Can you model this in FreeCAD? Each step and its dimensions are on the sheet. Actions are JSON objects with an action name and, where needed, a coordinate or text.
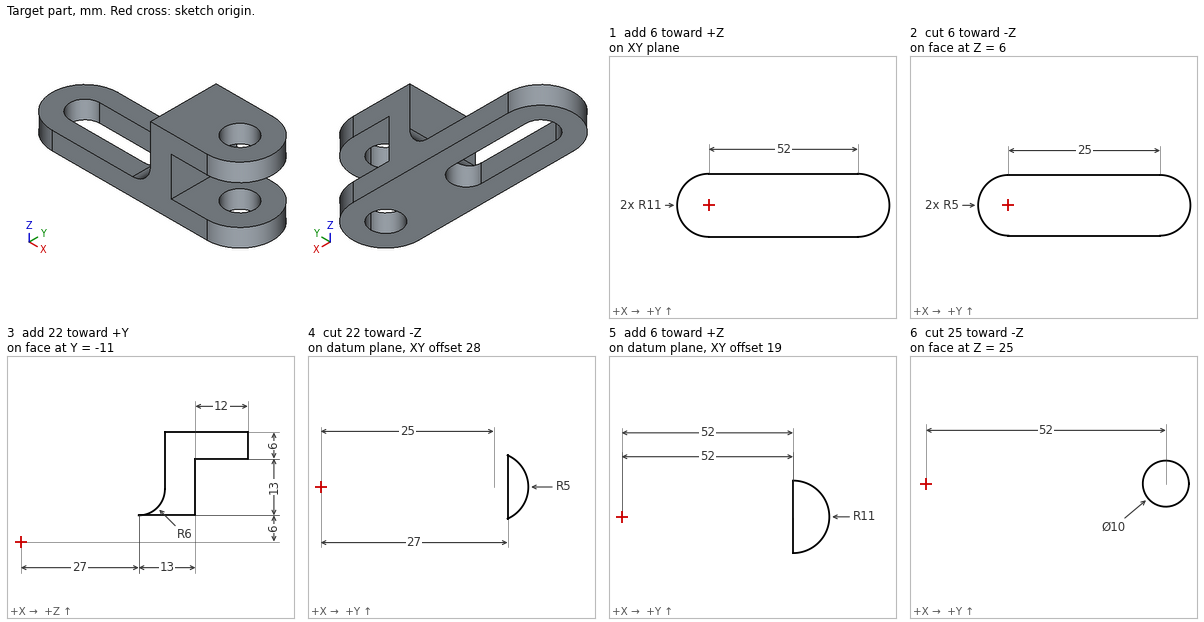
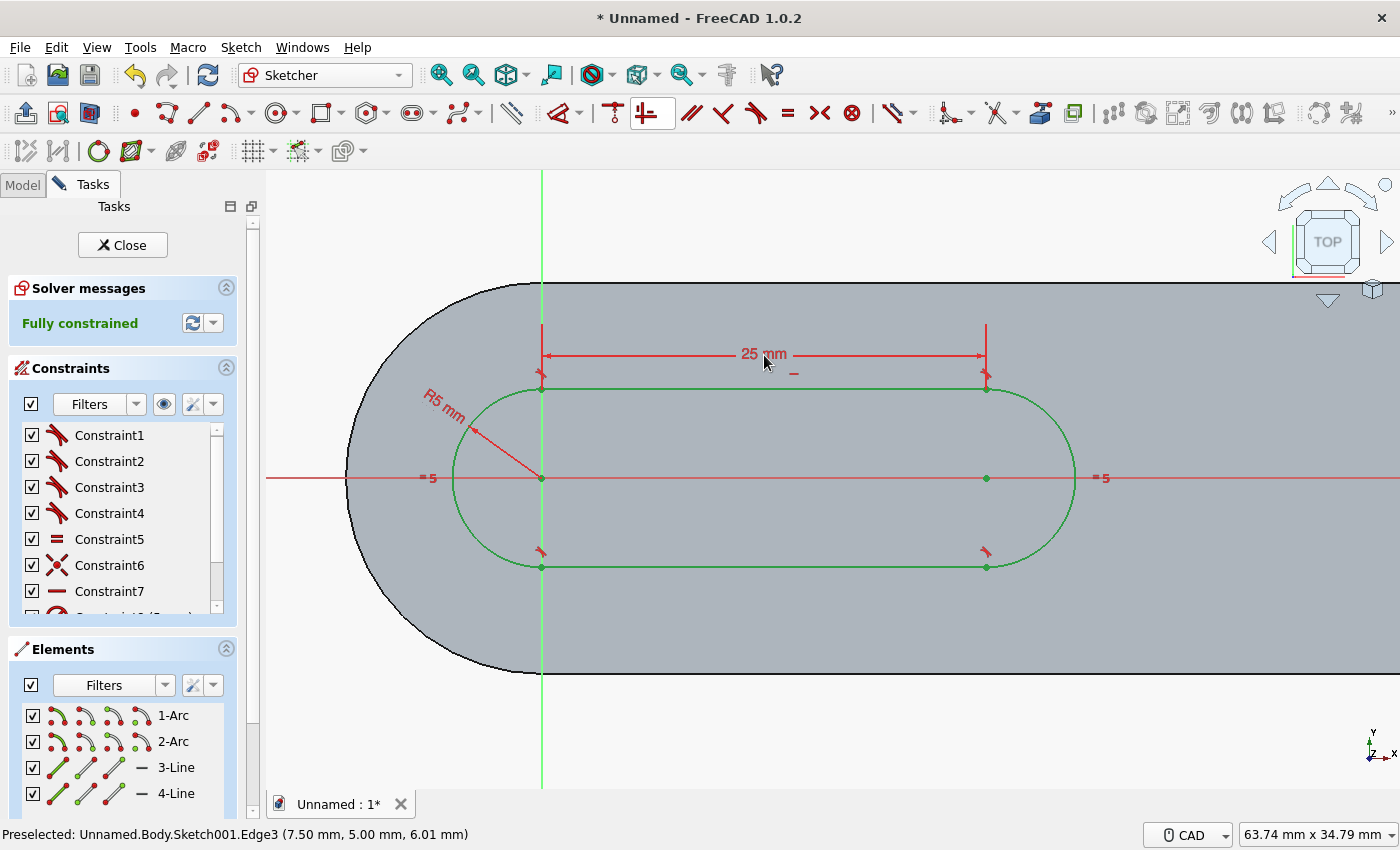
{"action": "left_click", "coordinate": [123, 245]}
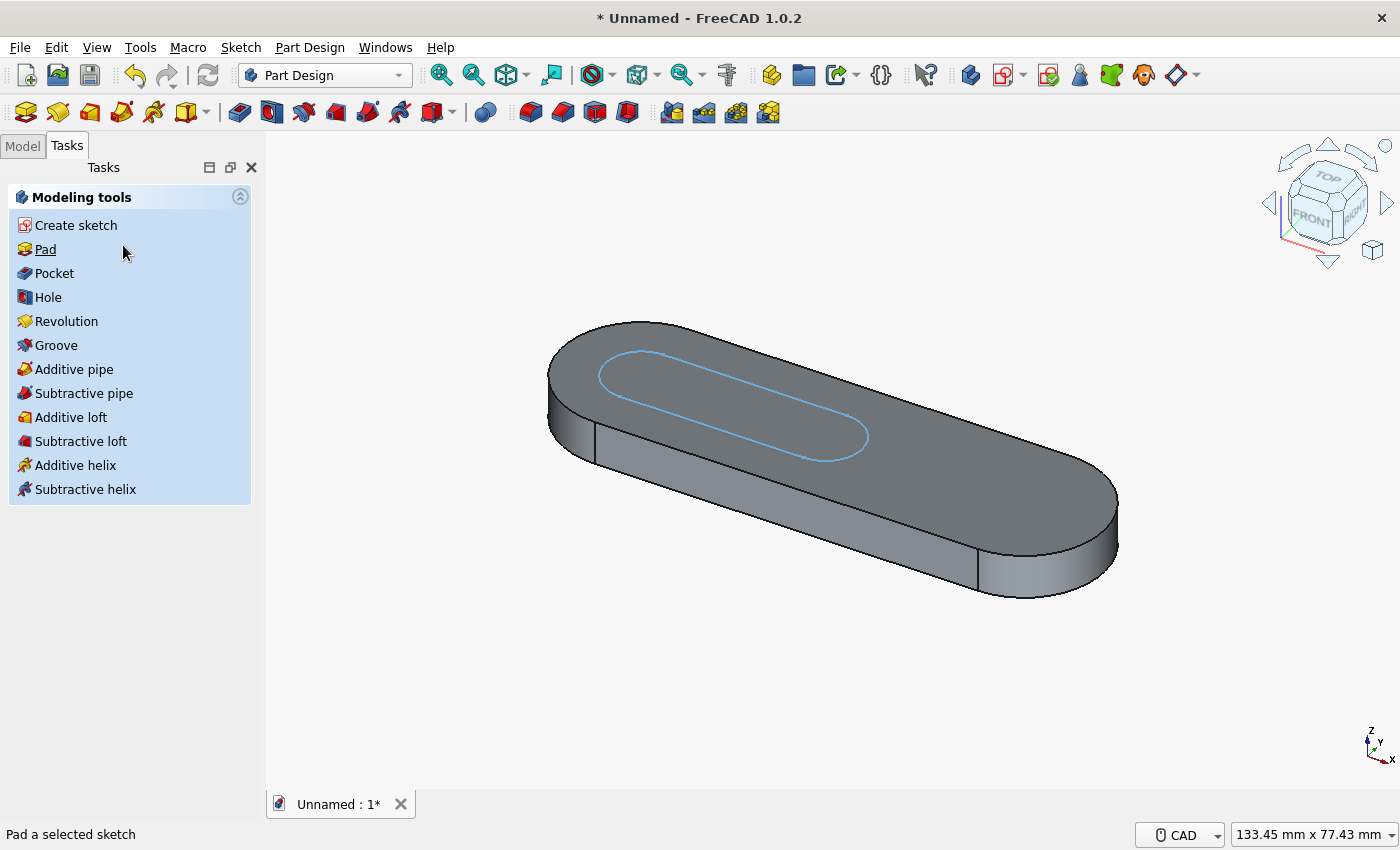
{"action": "left_click", "coordinate": [240, 112]}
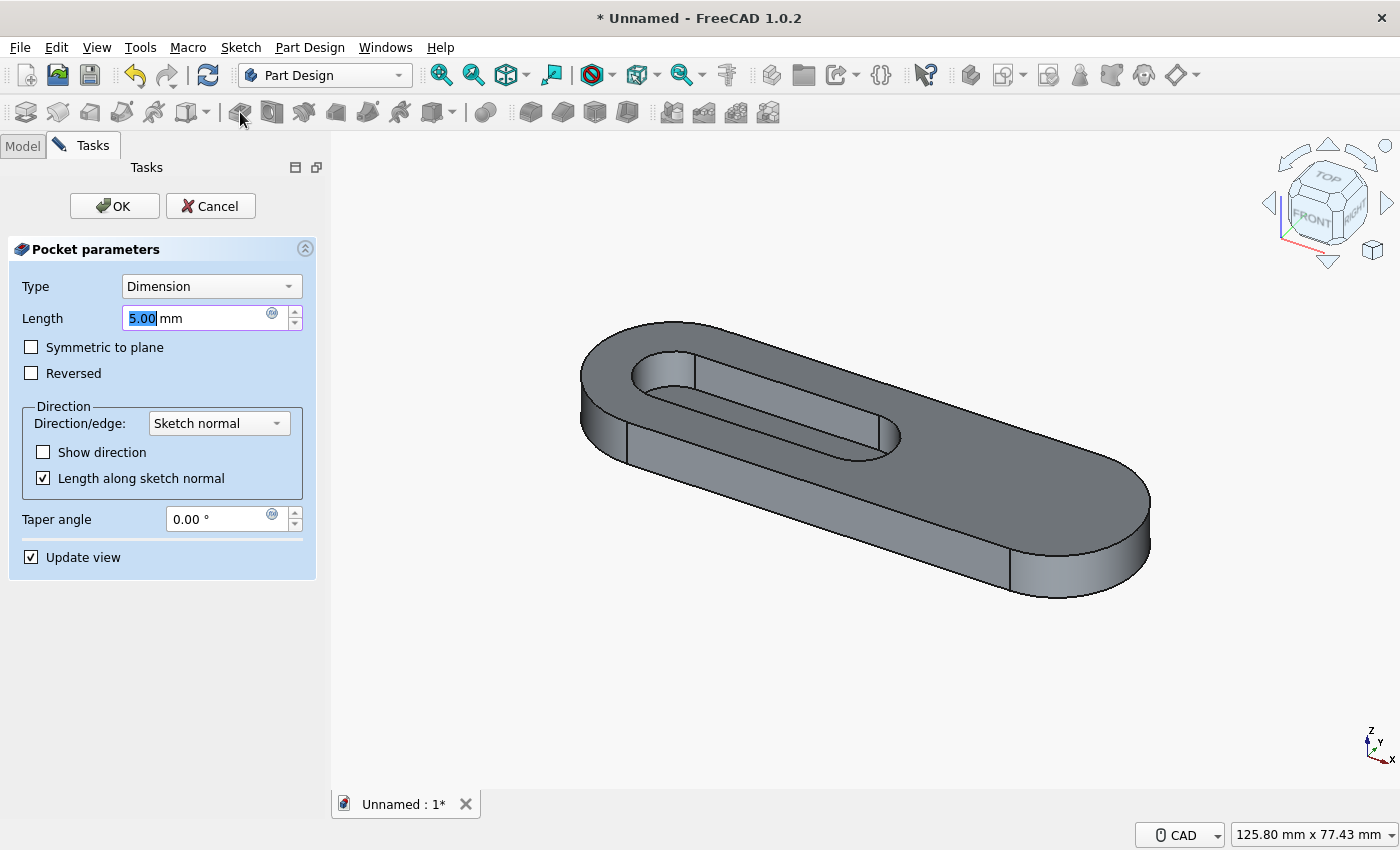
{"action": "type", "text": "6"}
{"action": "key", "text": "Tab"}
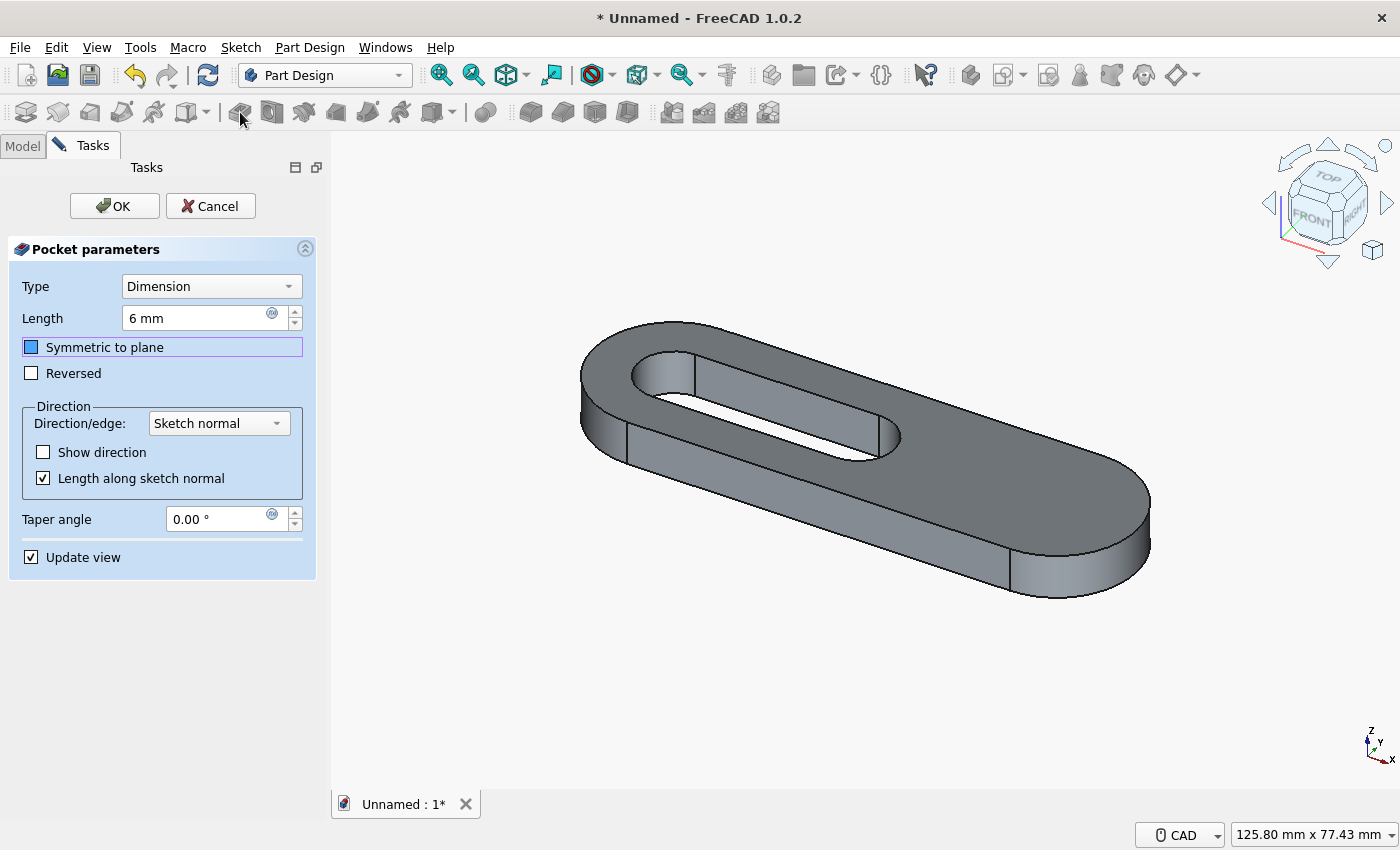
{"action": "left_click", "coordinate": [115, 206]}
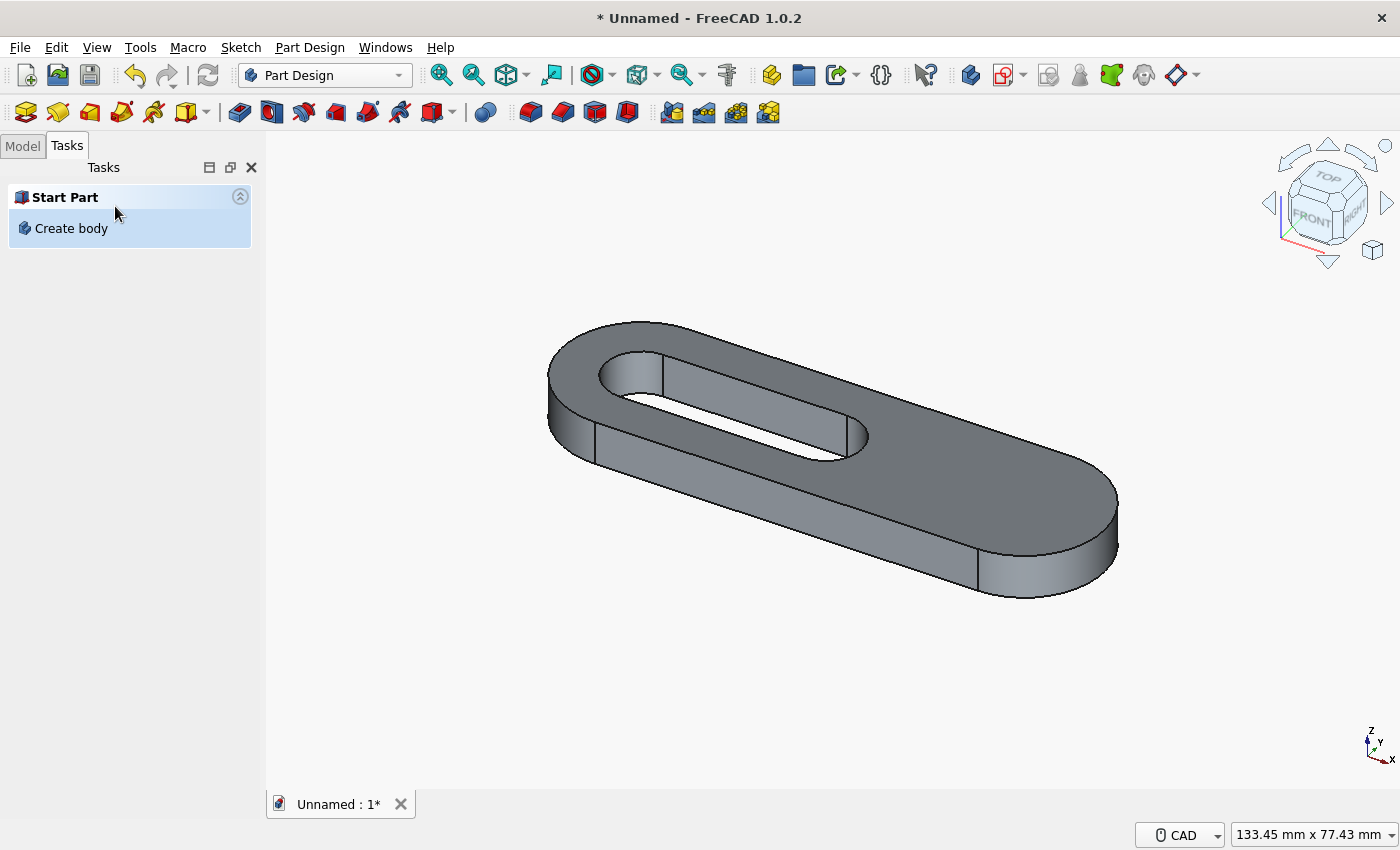
{"action": "left_click", "coordinate": [950, 560]}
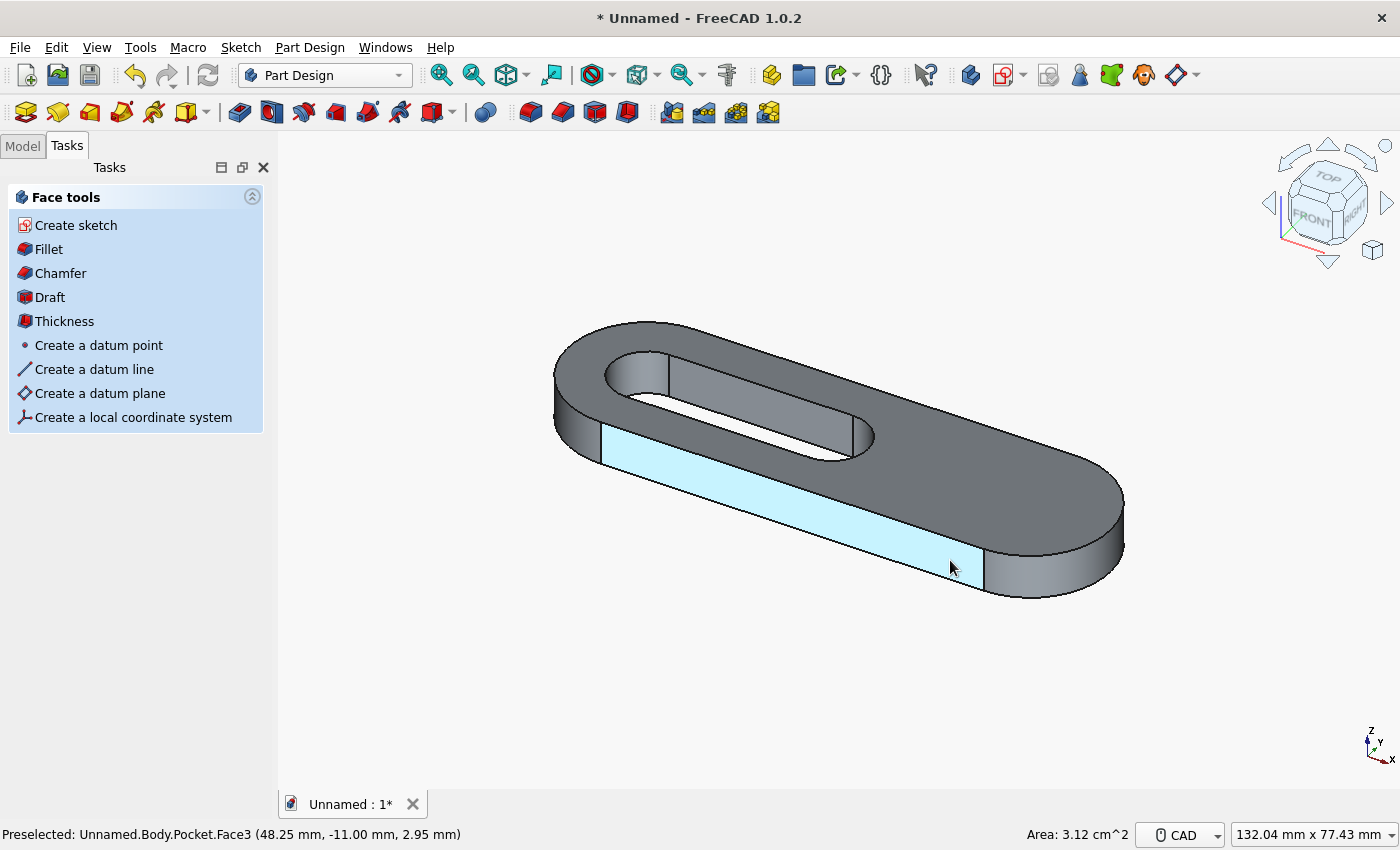
{"action": "left_click", "coordinate": [1004, 76]}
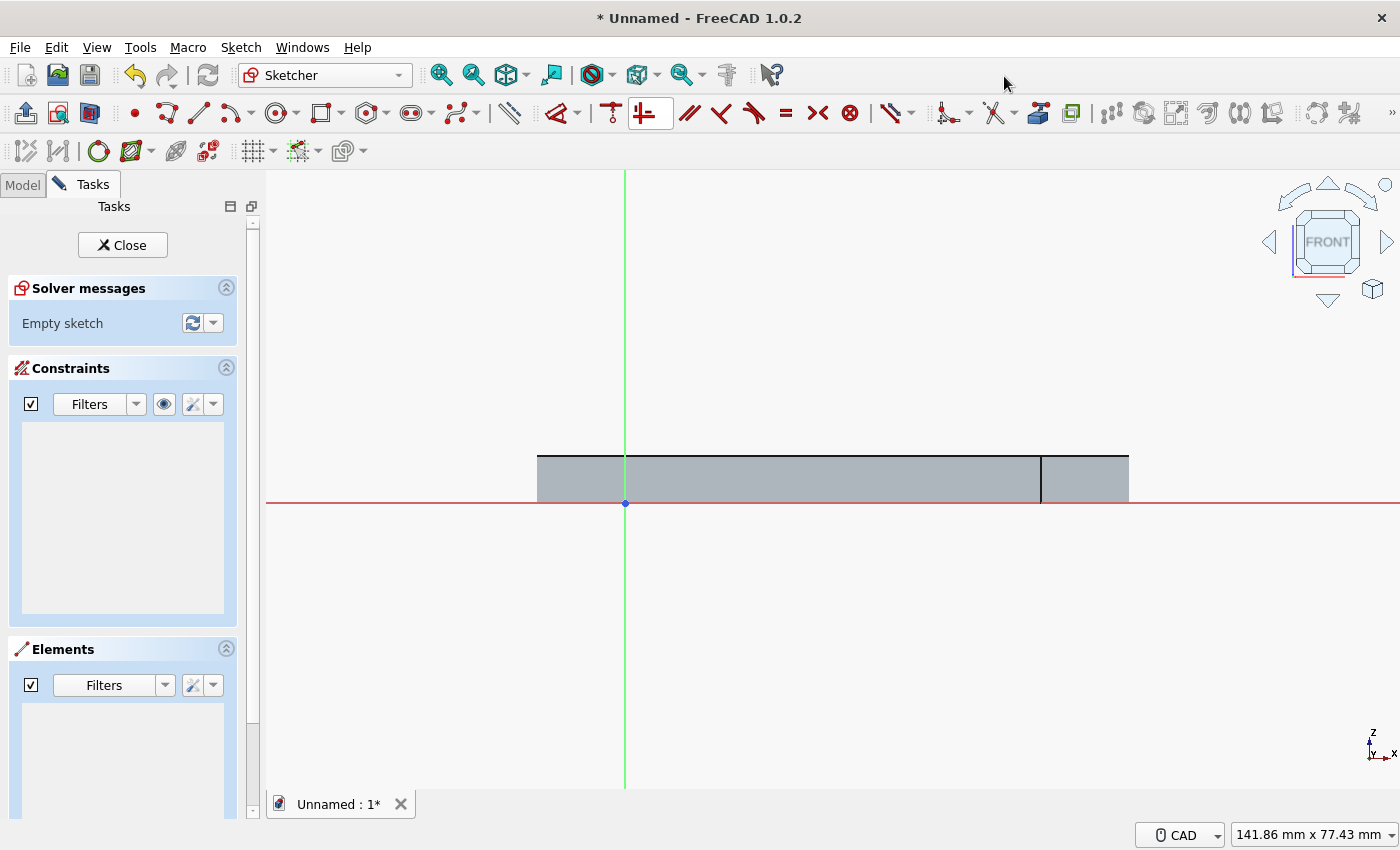
{"action": "scroll", "coordinate": [972, 249], "scroll_direction": "up", "scroll_amount": 2}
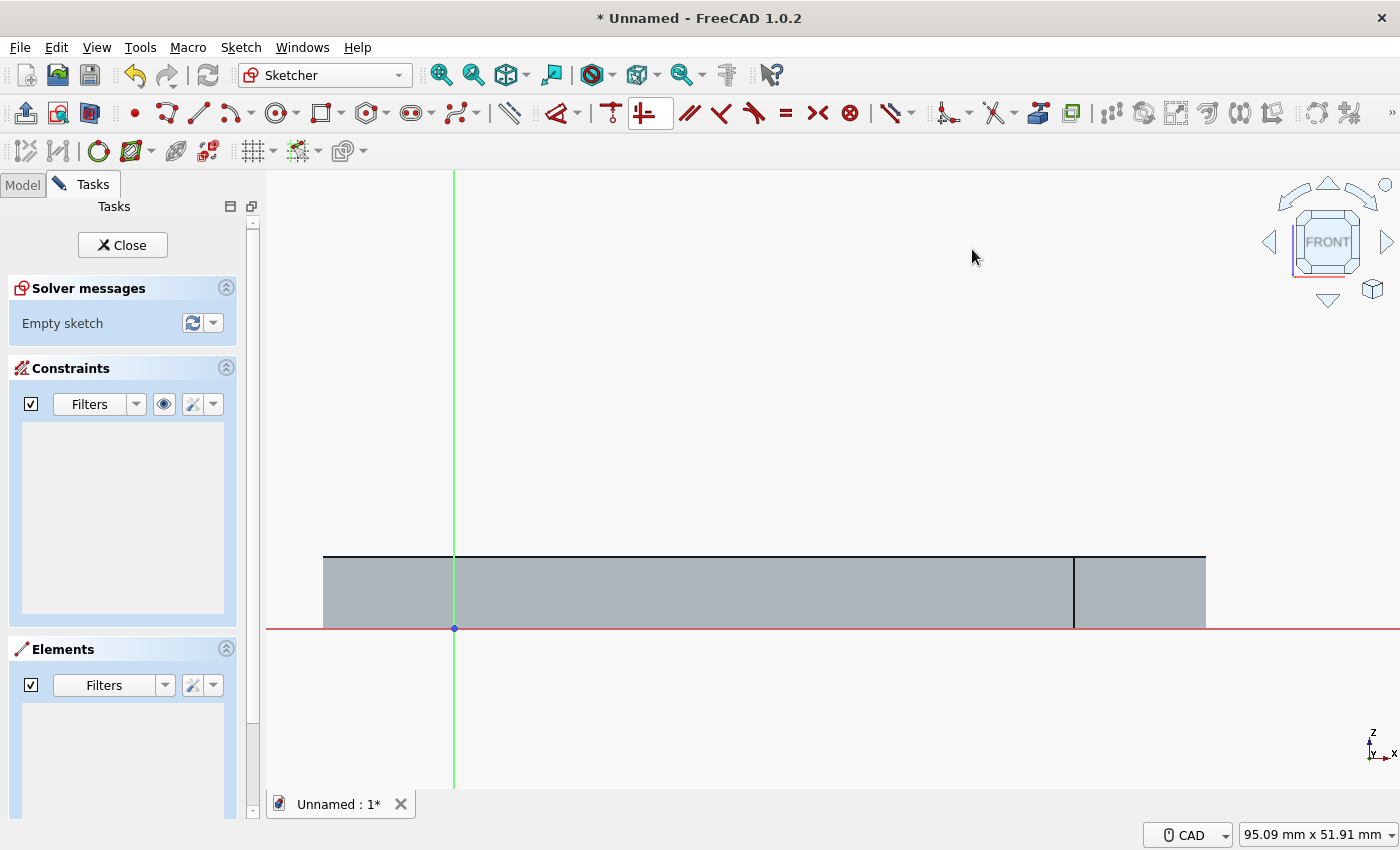
{"action": "left_click", "coordinate": [168, 114]}